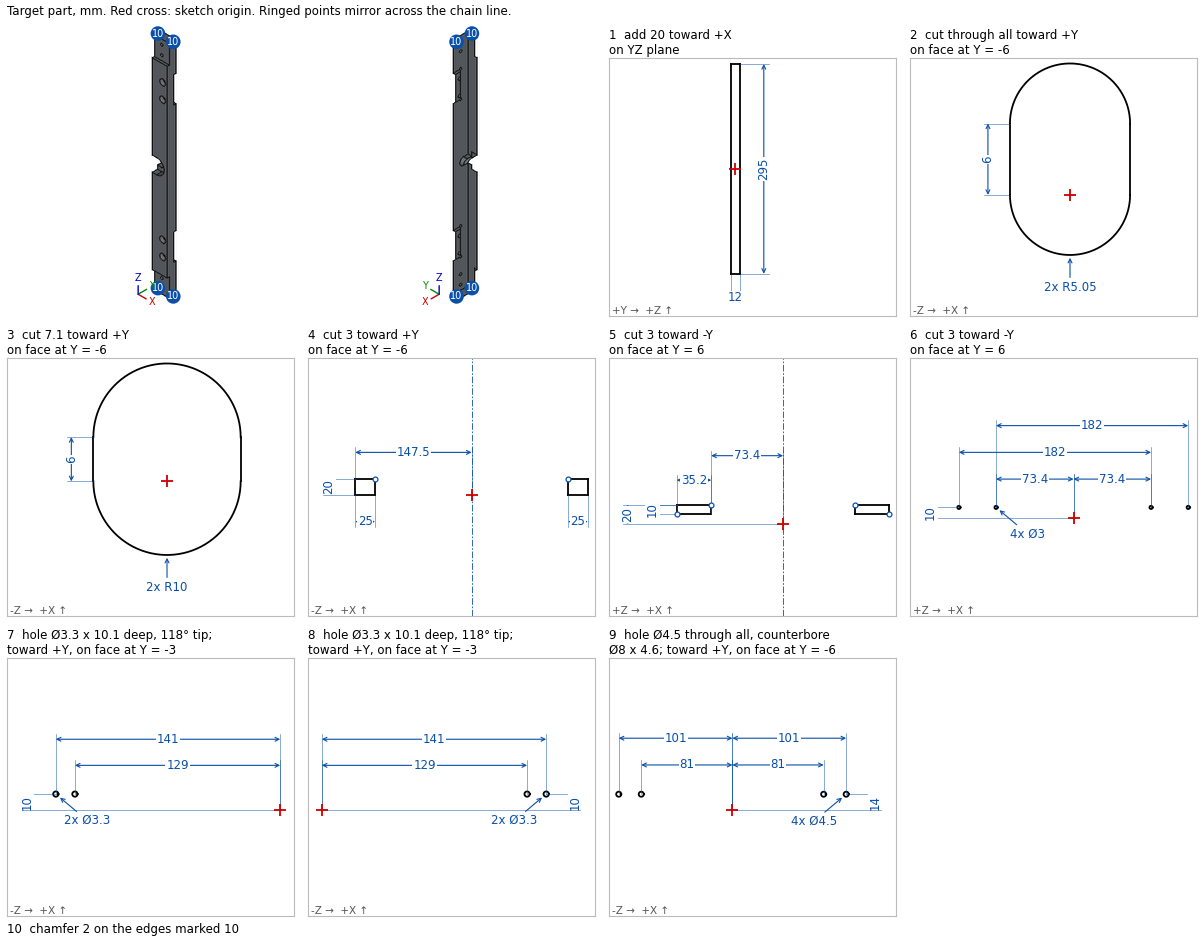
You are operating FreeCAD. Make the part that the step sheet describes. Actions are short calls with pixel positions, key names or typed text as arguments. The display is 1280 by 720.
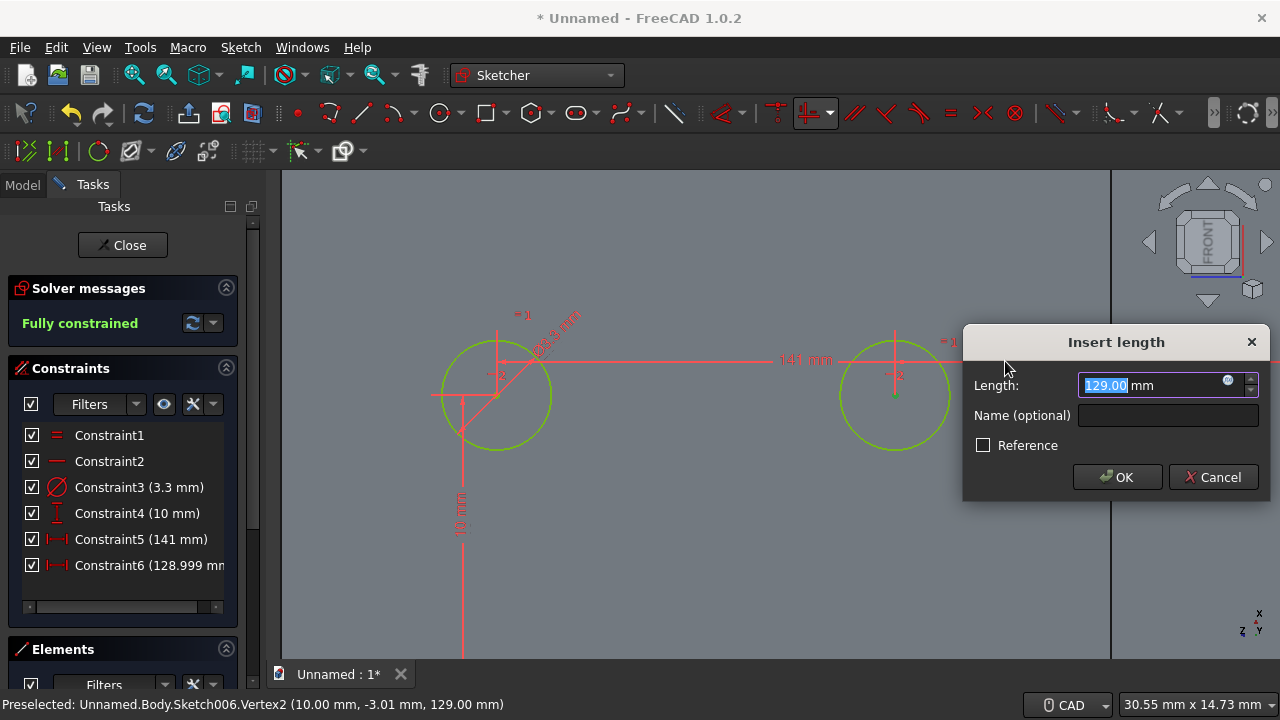
text(129)
key(Return)
key(Escape)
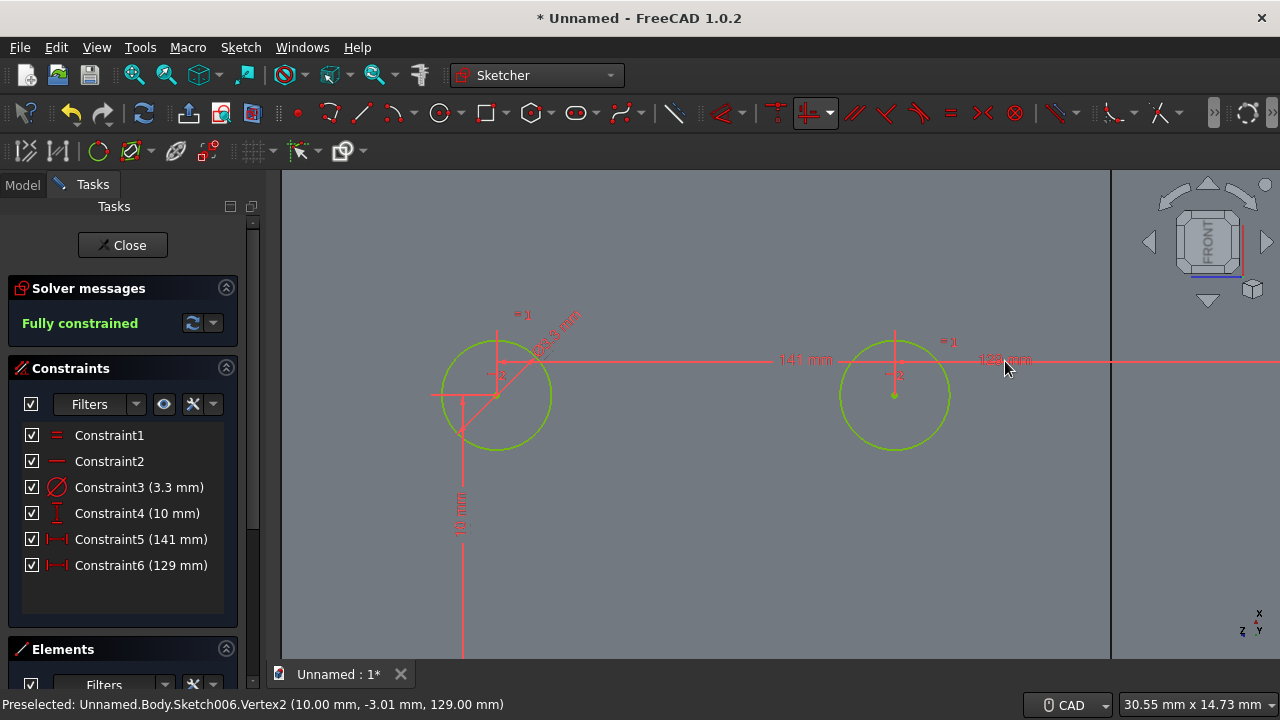
click(123, 245)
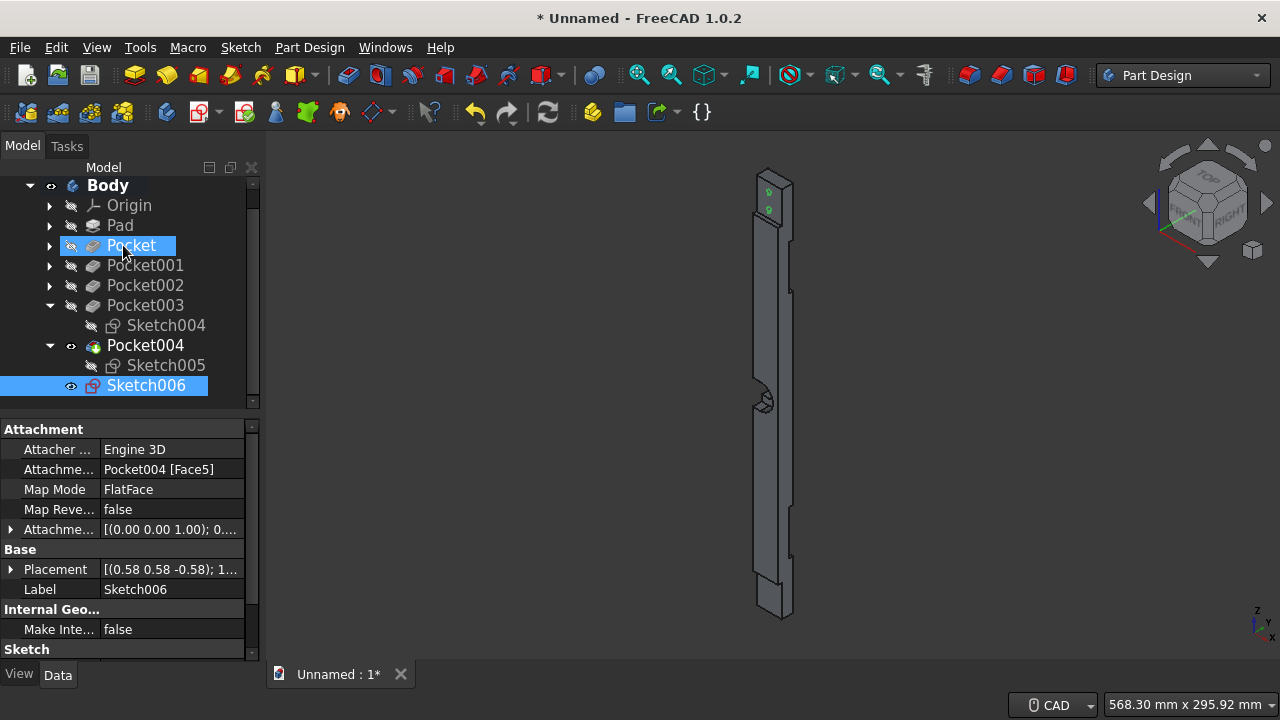
click(382, 76)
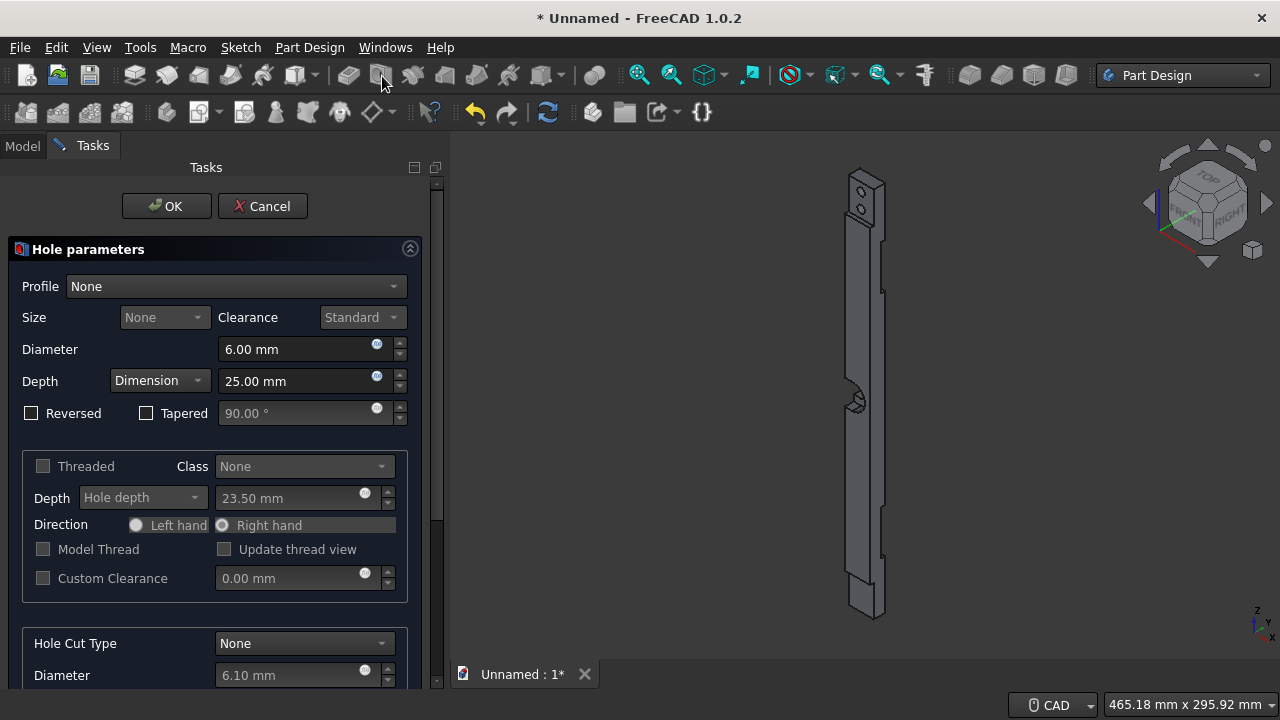
triple_click(305, 349)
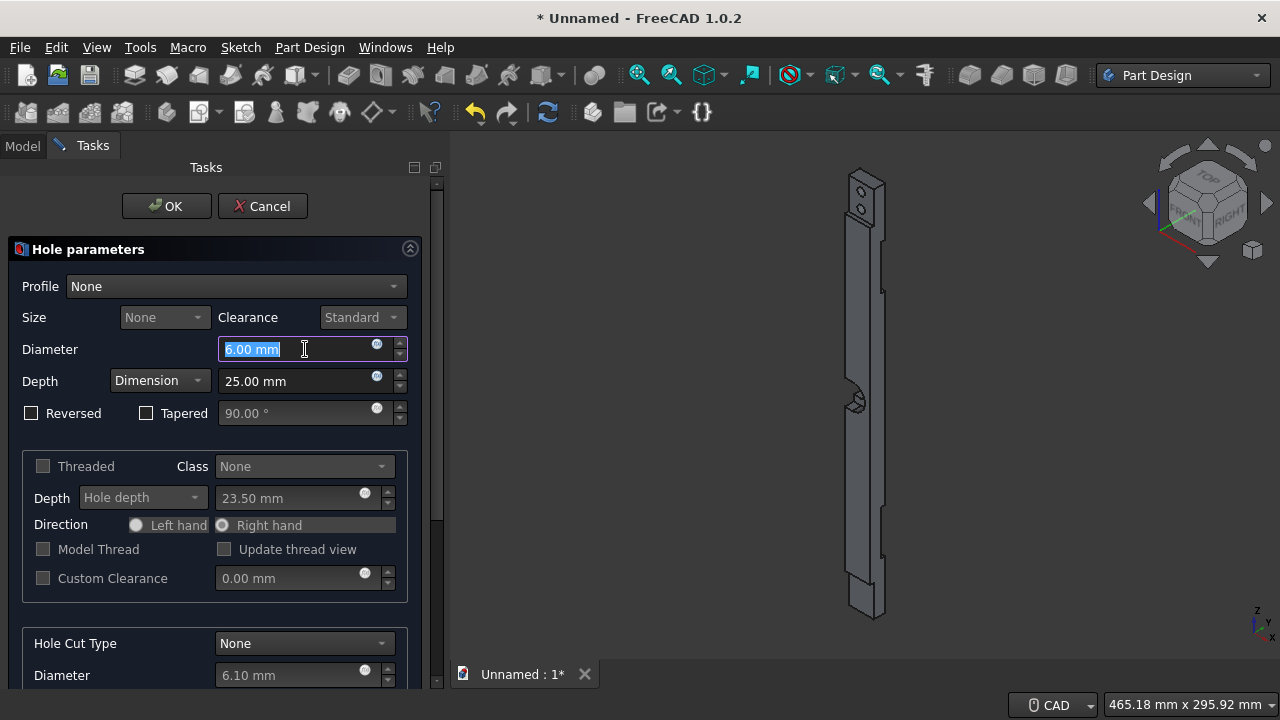
text(3.3)
key(Tab)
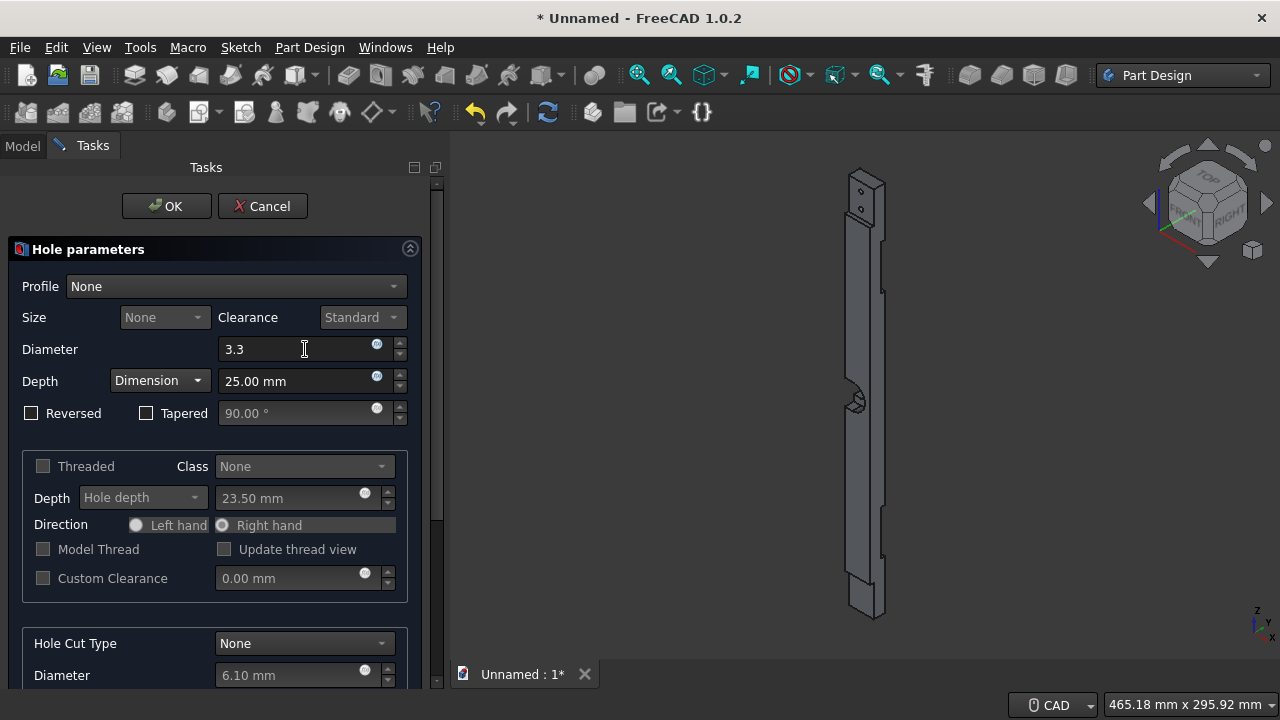
triple_click(305, 381)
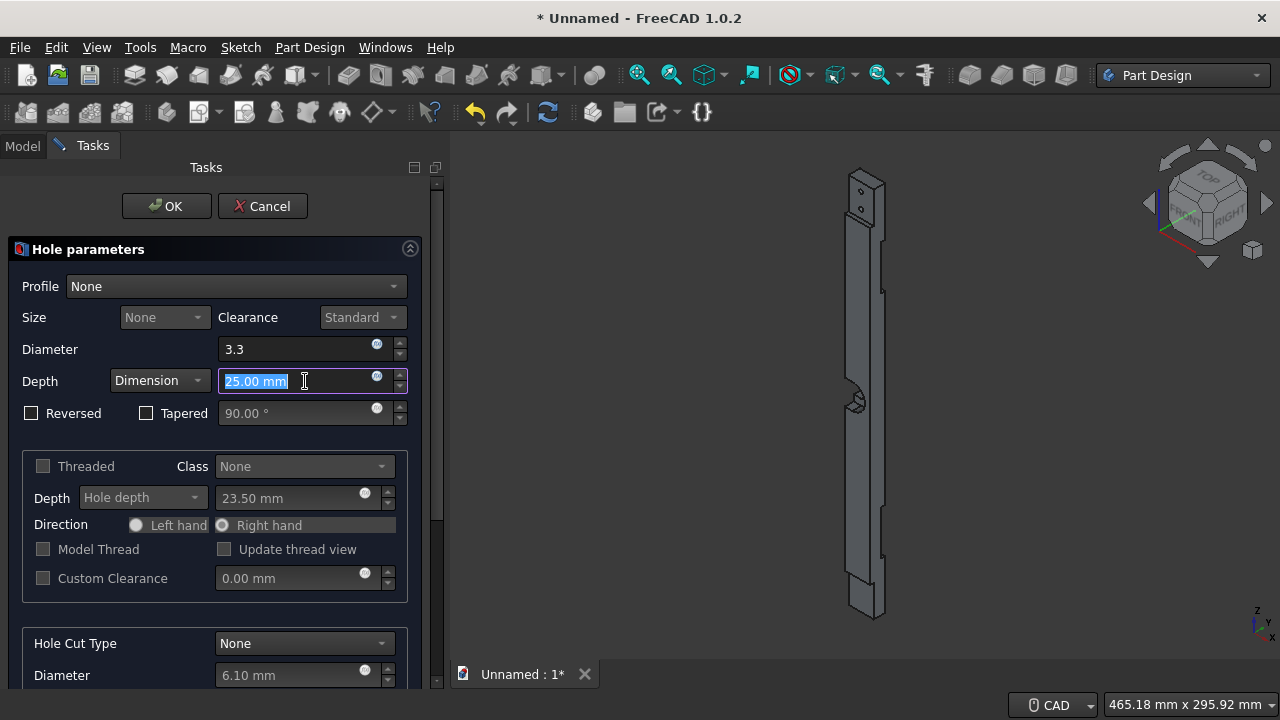
text(10.1)
key(Tab)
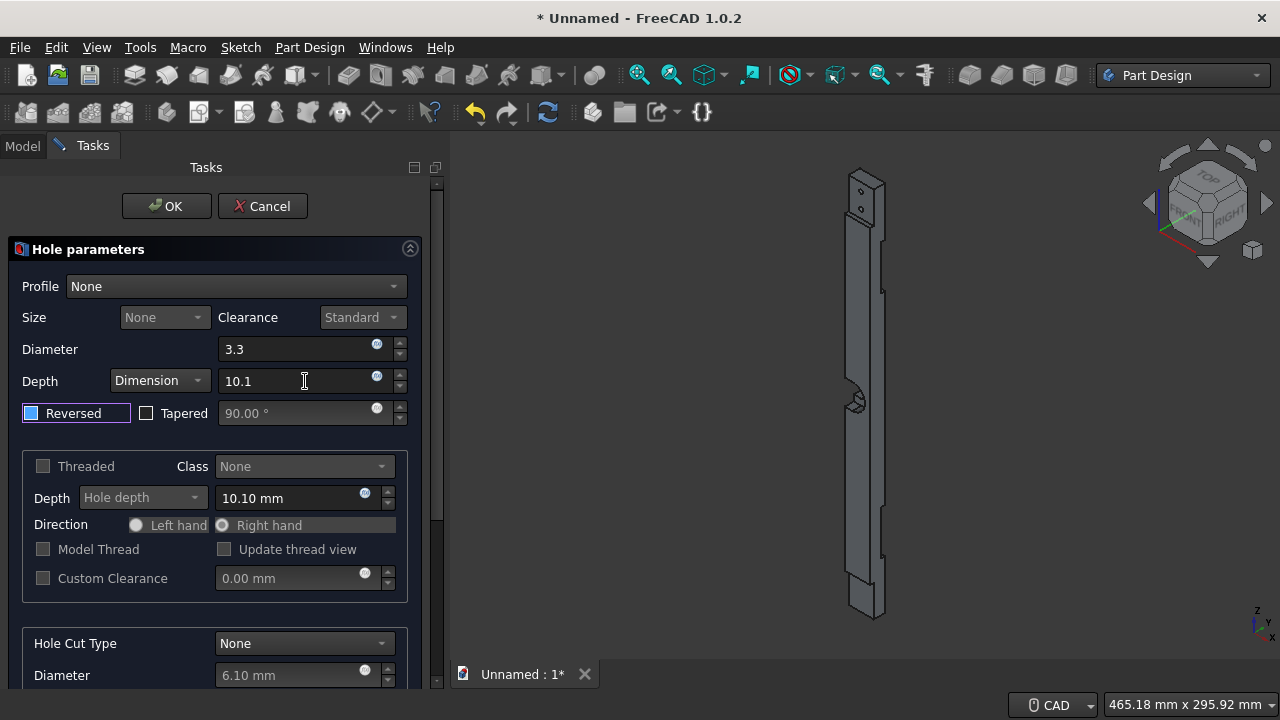
click(167, 206)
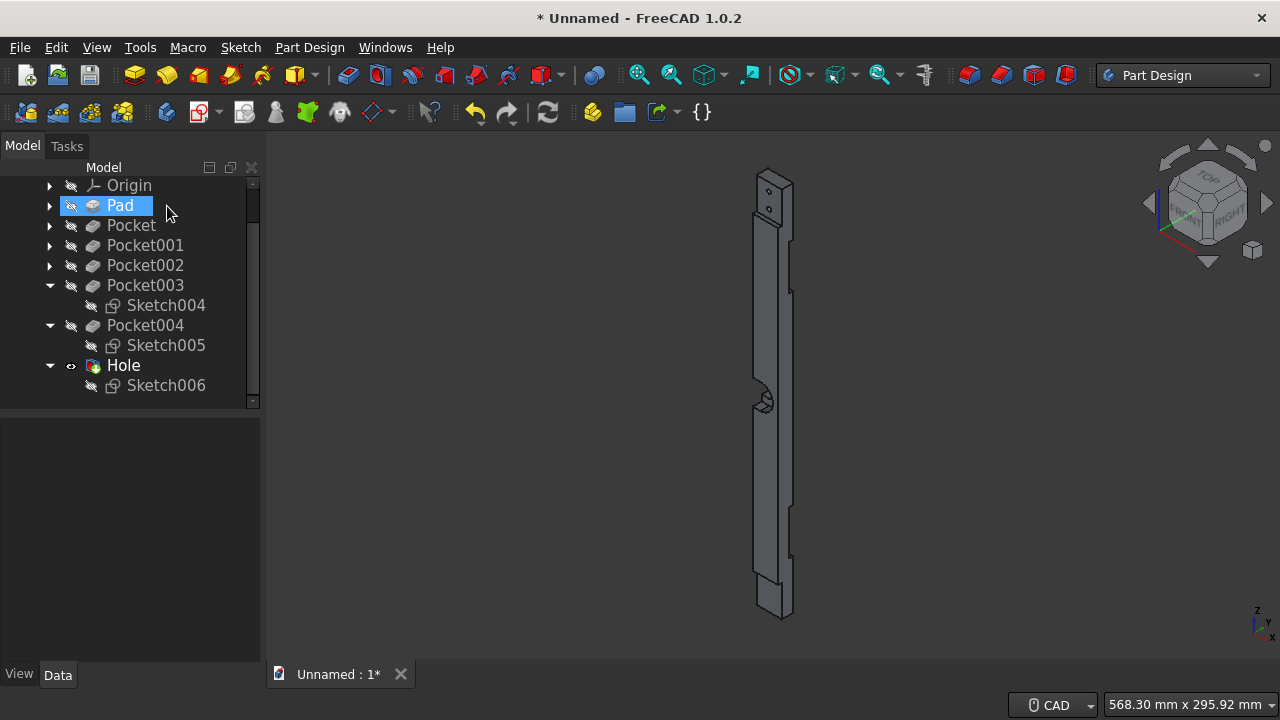
click(769, 593)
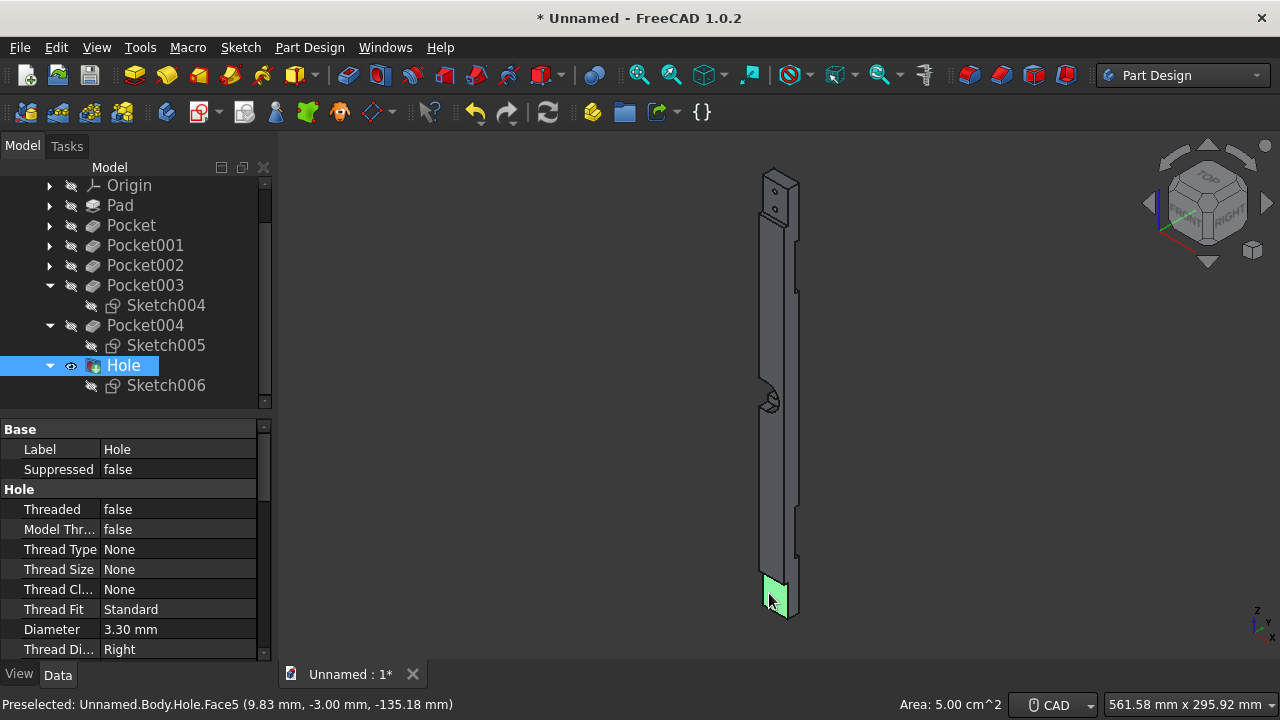
click(200, 112)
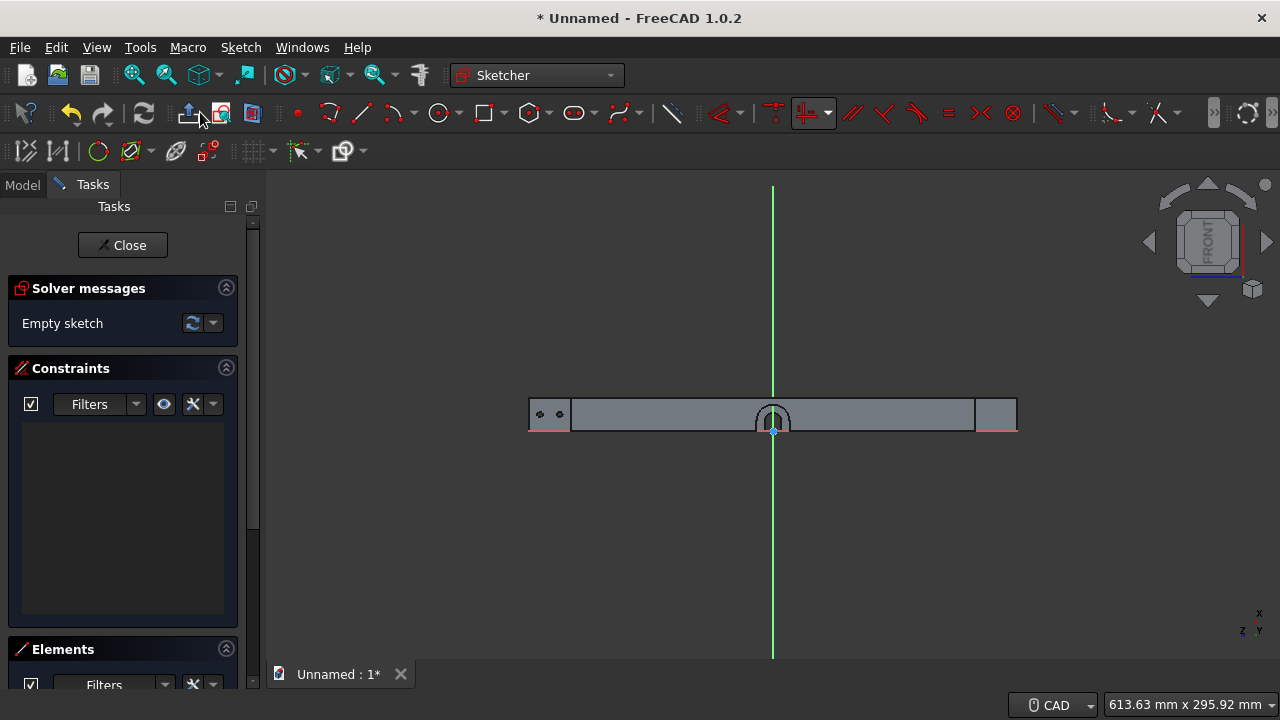
scroll(1011, 415, up, 15)